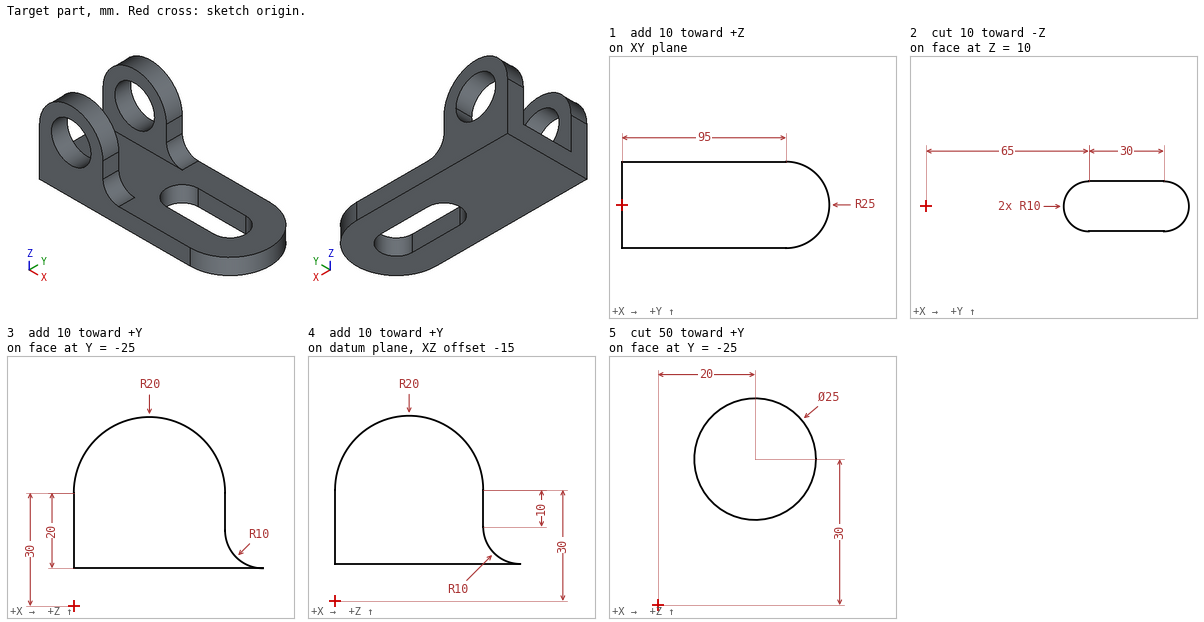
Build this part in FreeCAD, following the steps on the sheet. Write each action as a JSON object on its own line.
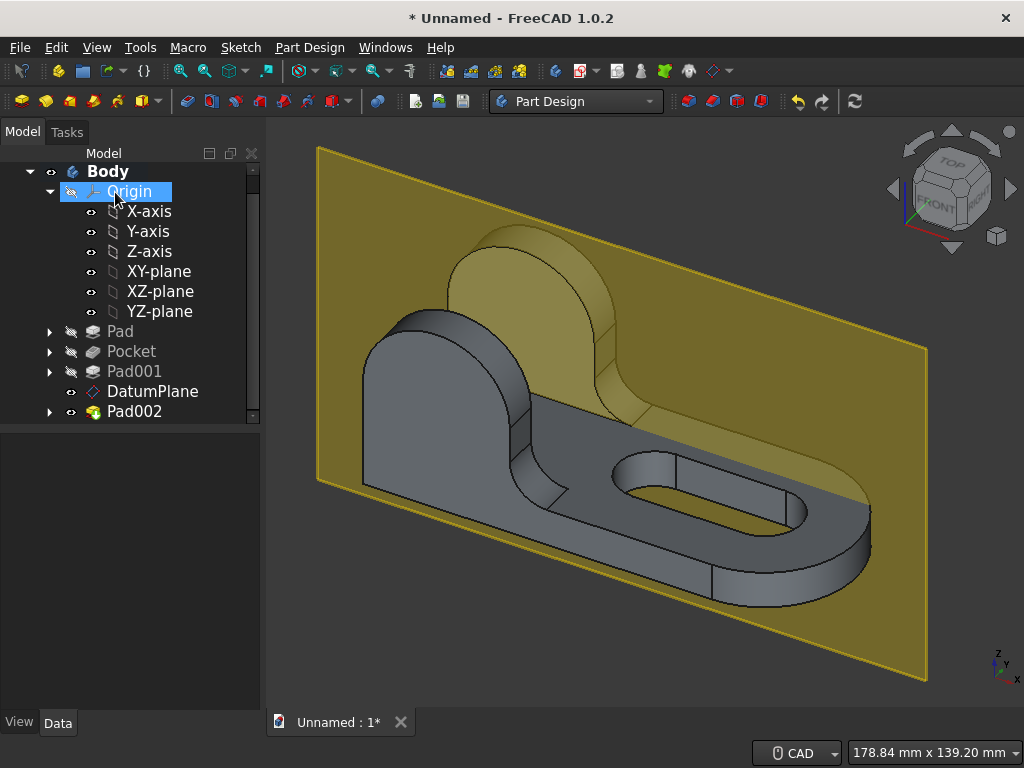
{"action": "left_click", "coordinate": [116, 392]}
{"action": "key", "text": "space"}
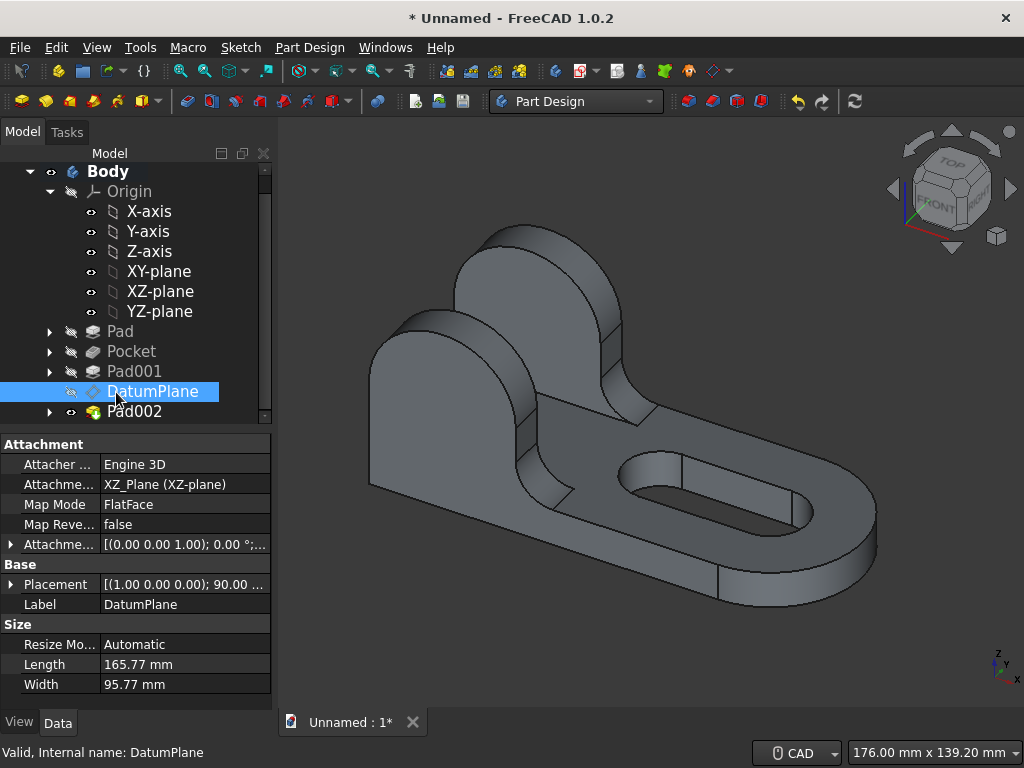
{"action": "left_click", "coordinate": [444, 421]}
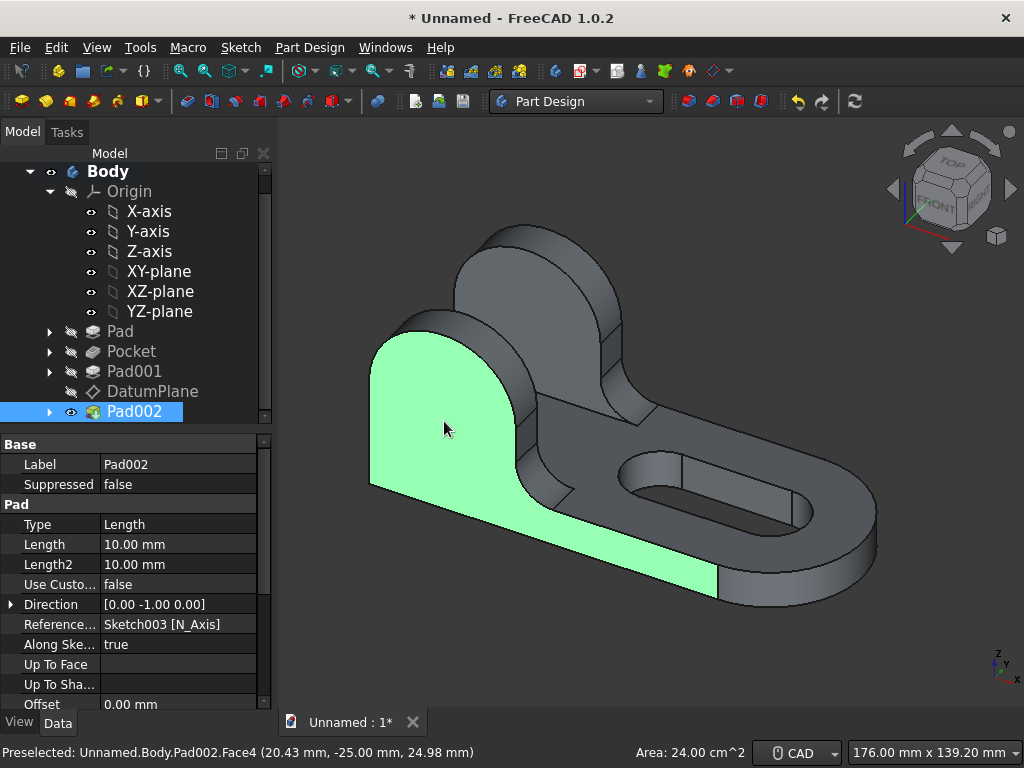
{"action": "left_click", "coordinate": [580, 72]}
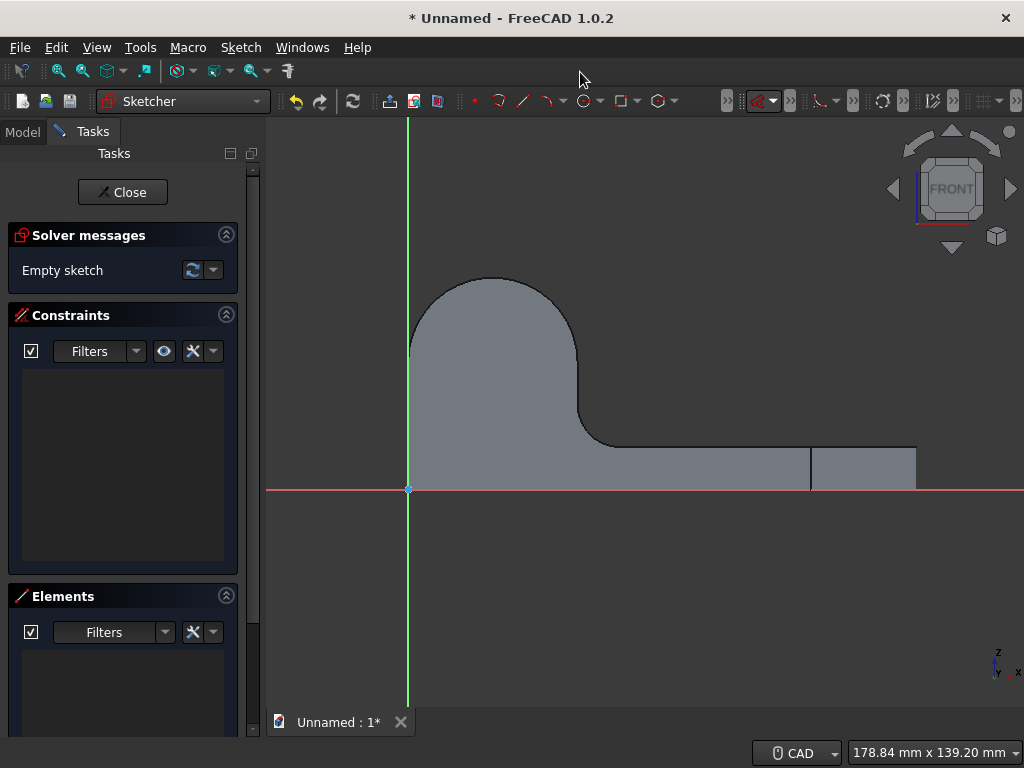
{"action": "scroll", "coordinate": [396, 389], "scroll_direction": "up", "scroll_amount": 4}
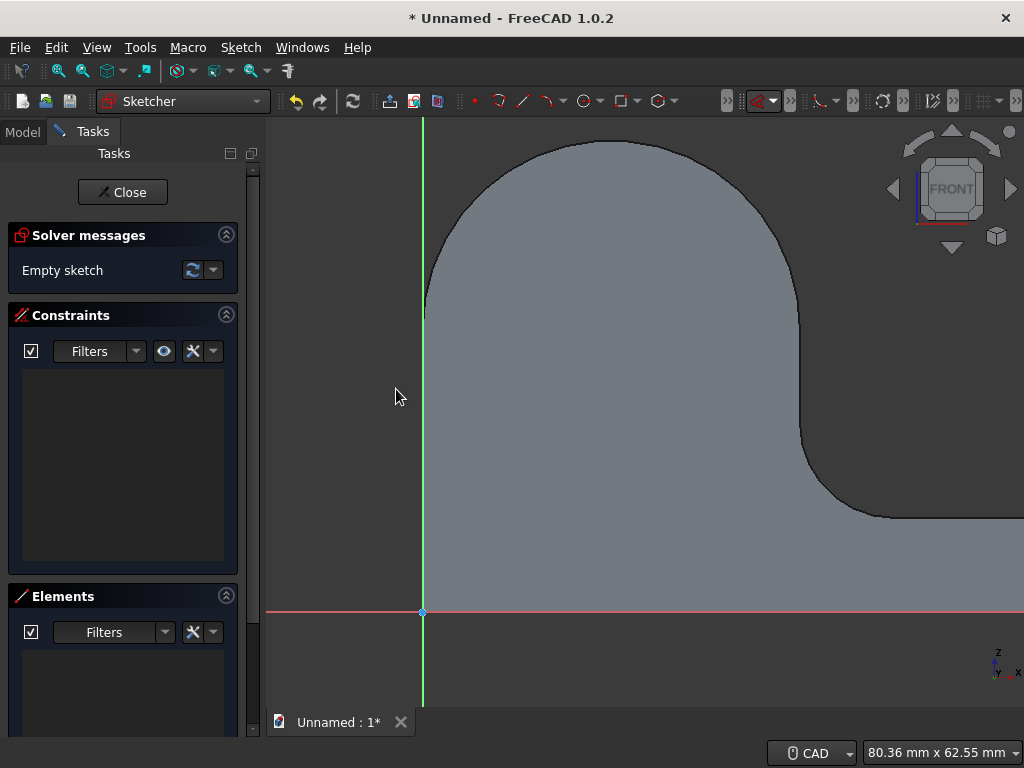
{"action": "left_click", "coordinate": [584, 102]}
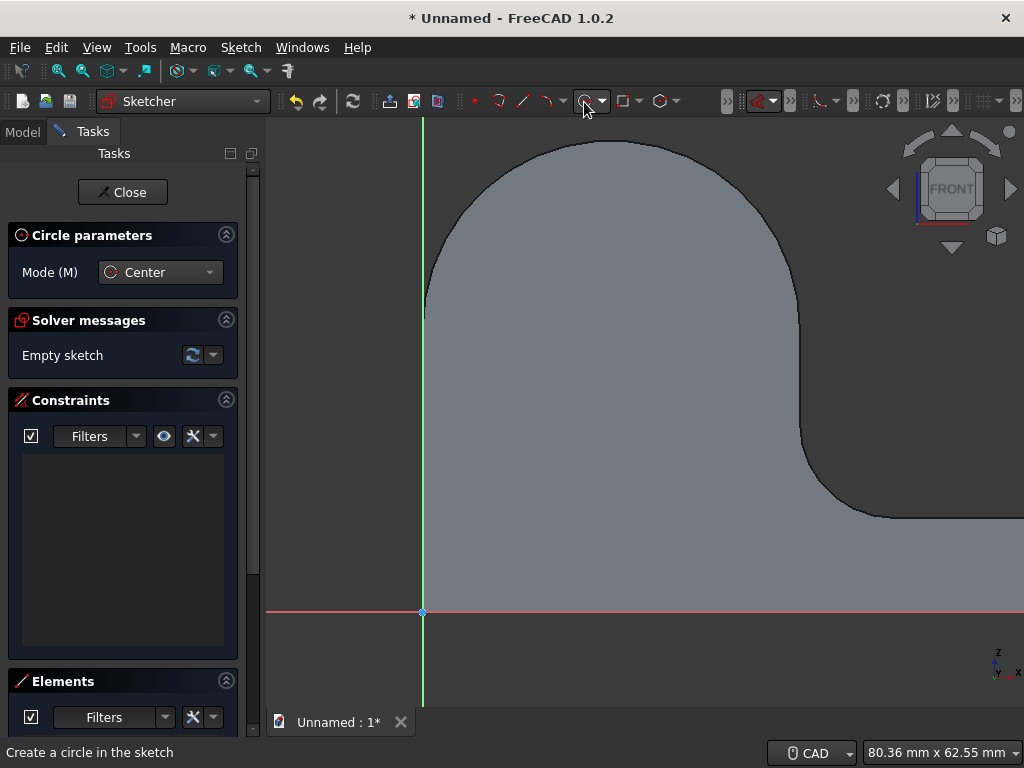
{"action": "left_click", "coordinate": [611, 329]}
{"action": "left_click", "coordinate": [695, 246]}
{"action": "key", "text": "Escape"}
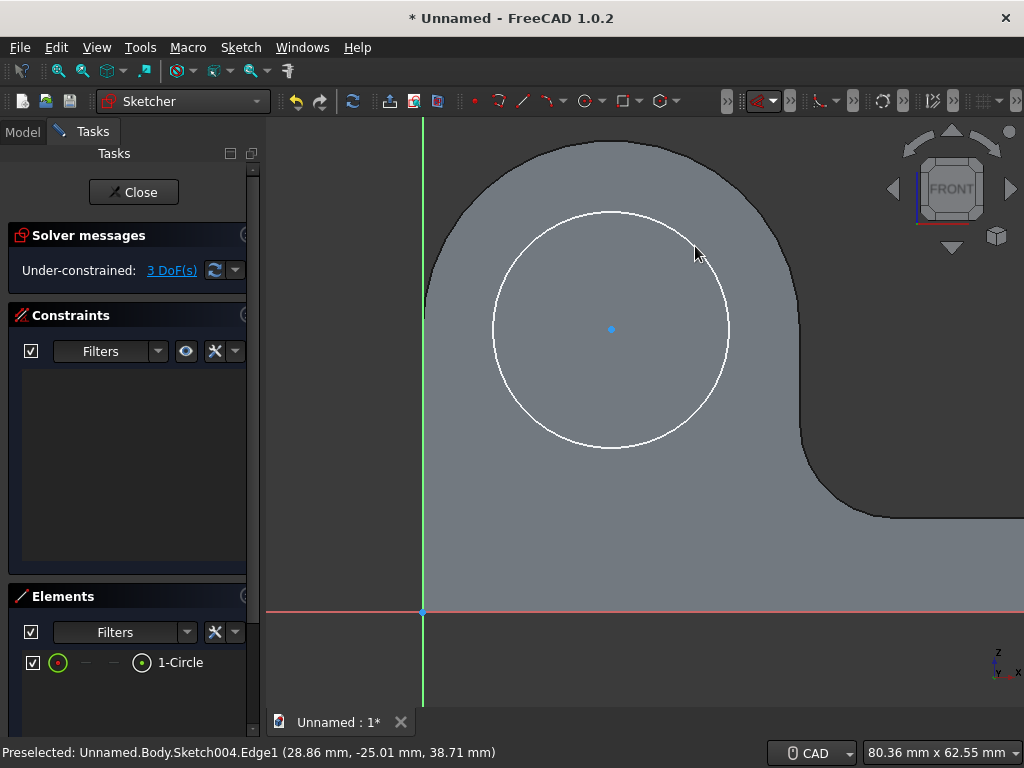
{"action": "left_click", "coordinate": [694, 246]}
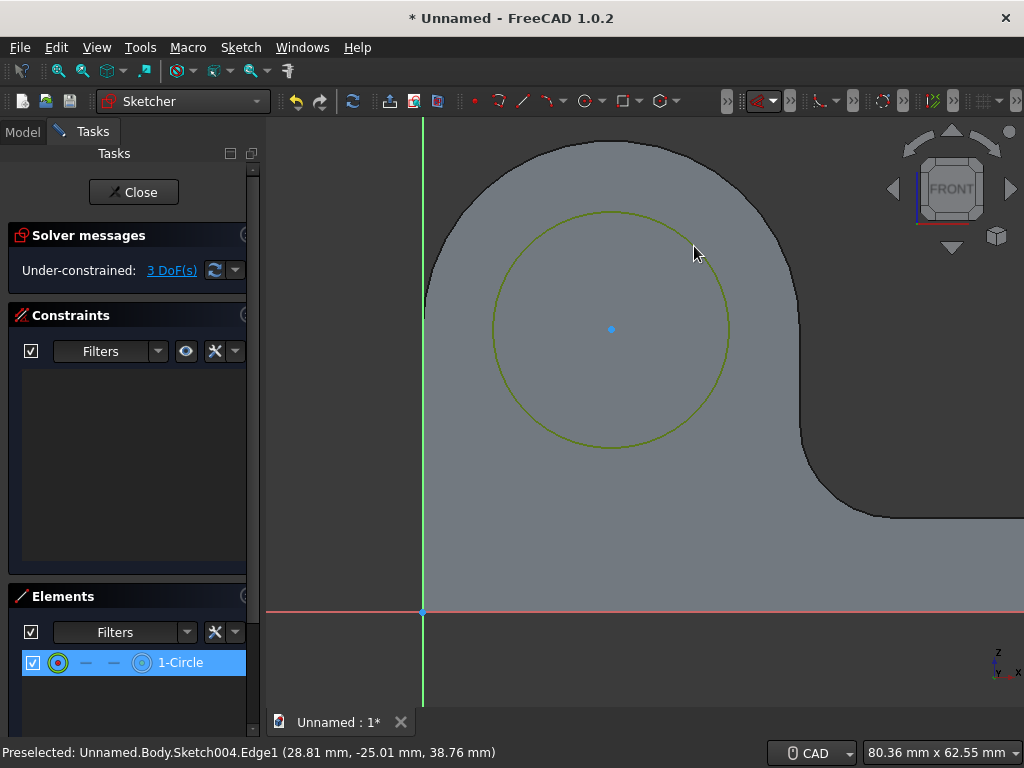
{"action": "key", "text": "k o"}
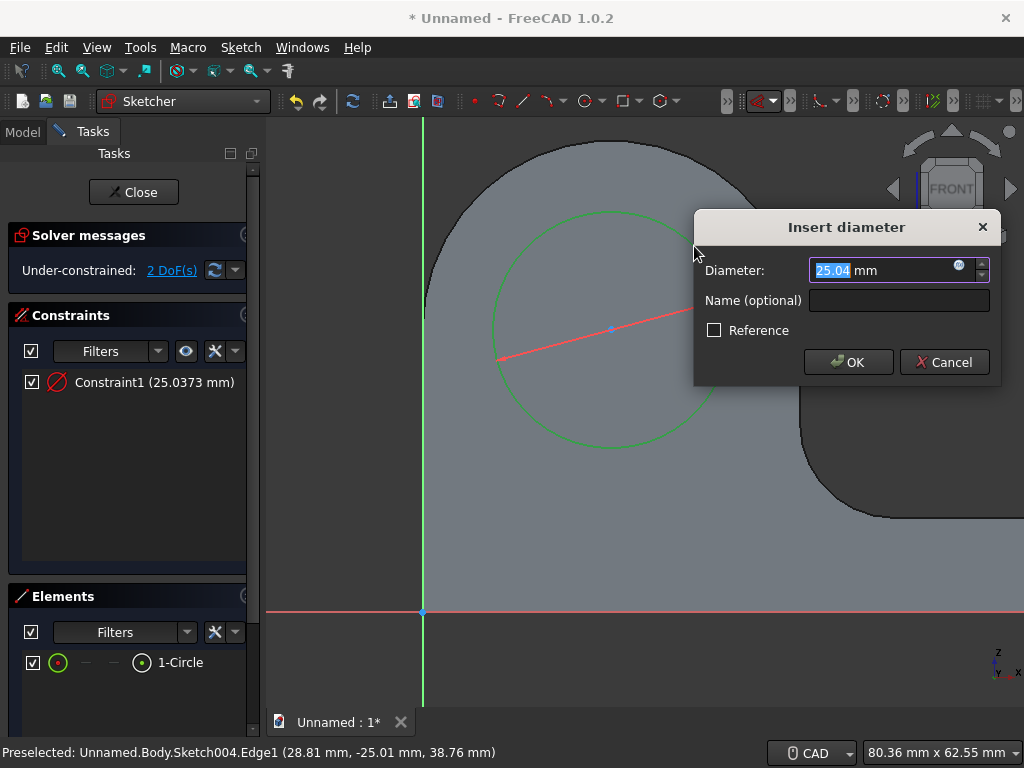
{"action": "type", "text": "25"}
{"action": "key", "text": "Return"}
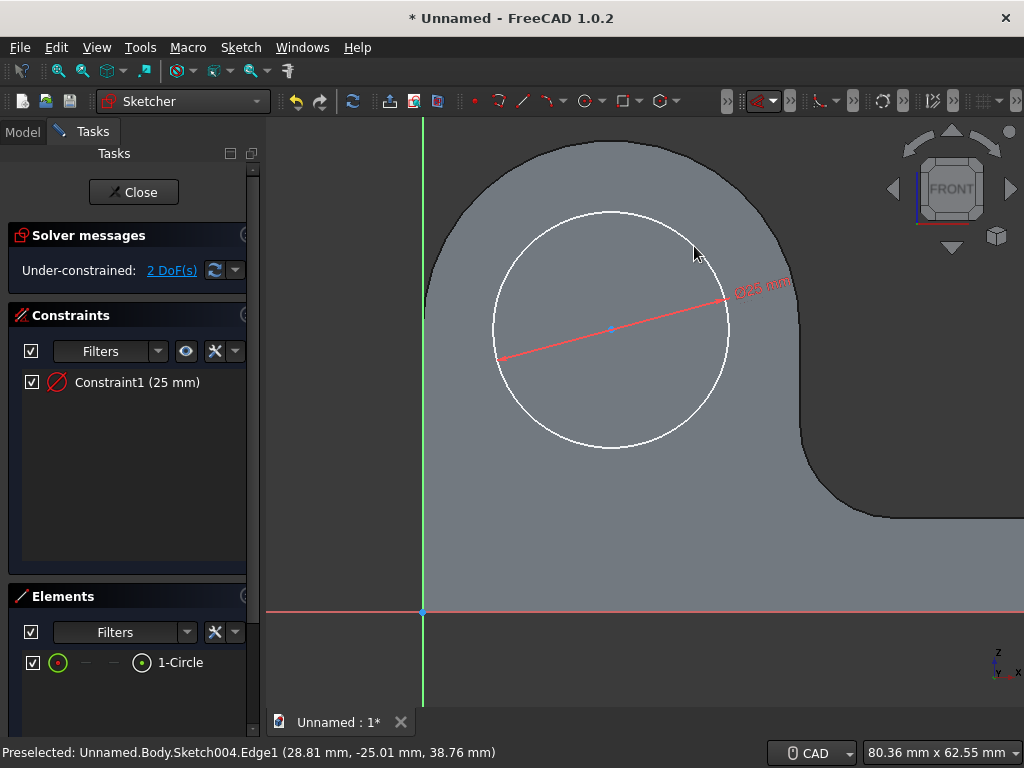
{"action": "left_click", "coordinate": [611, 330]}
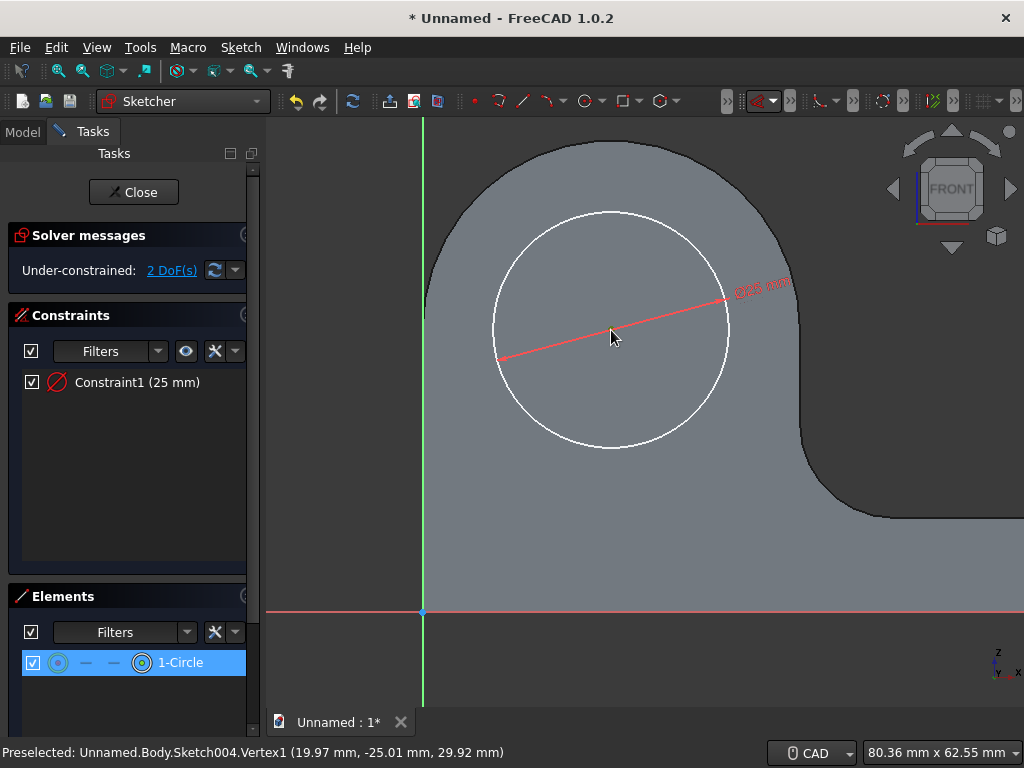
{"action": "left_click", "coordinate": [776, 102]}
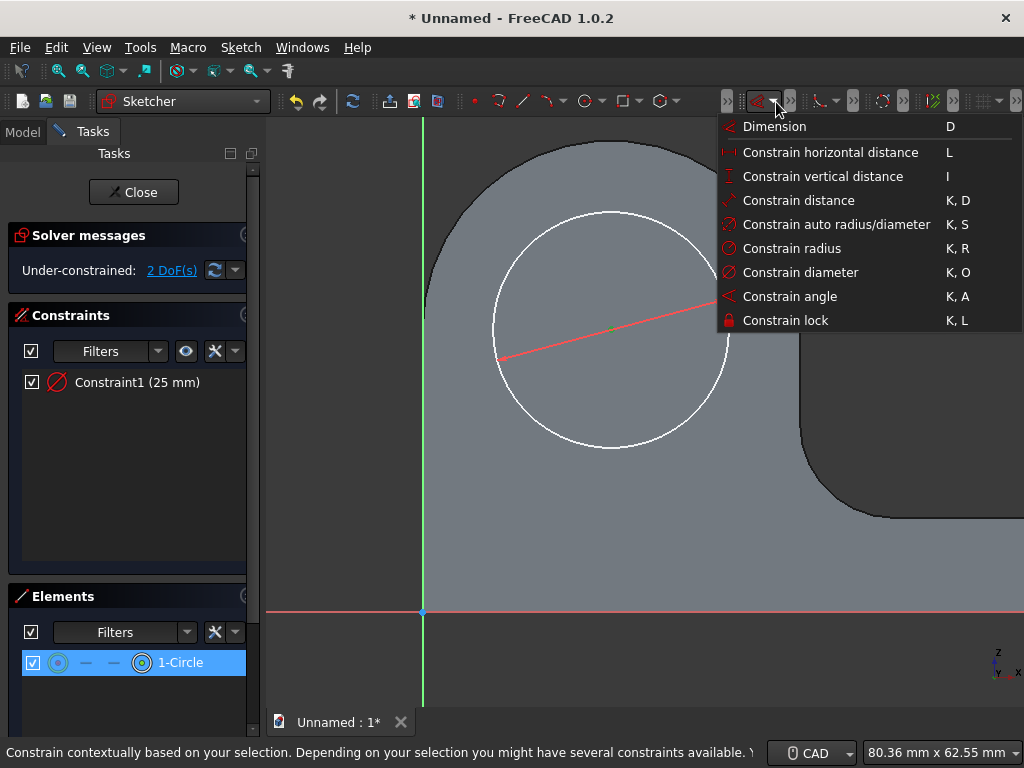
{"action": "left_click", "coordinate": [870, 152]}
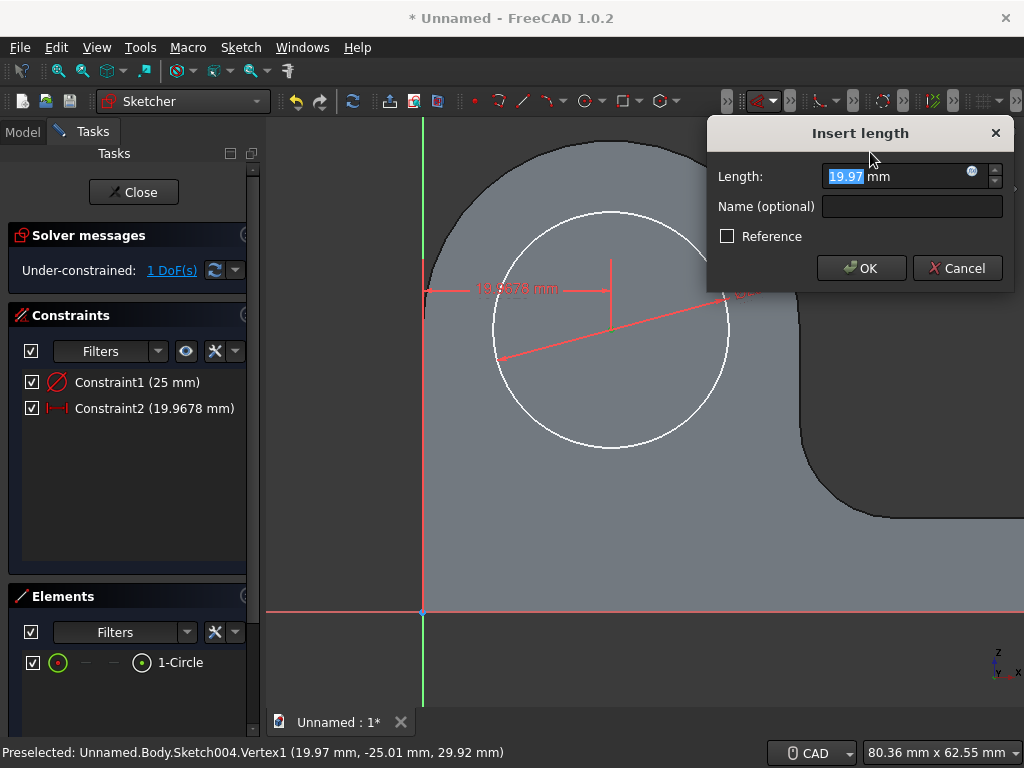
{"action": "type", "text": "20"}
{"action": "key", "text": "Return"}